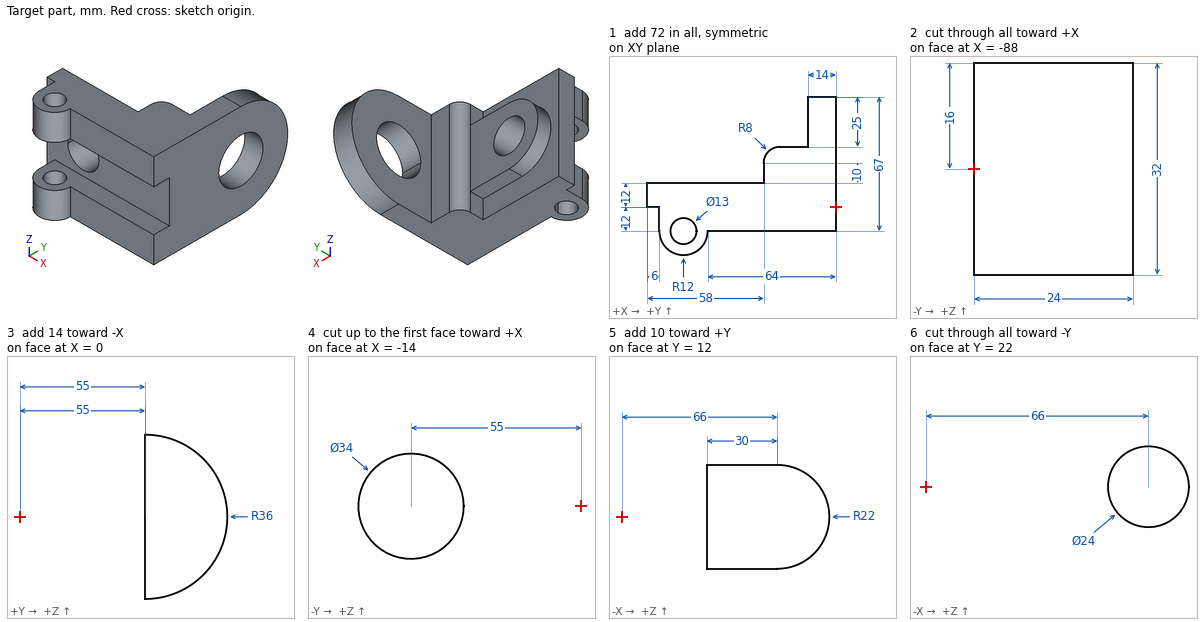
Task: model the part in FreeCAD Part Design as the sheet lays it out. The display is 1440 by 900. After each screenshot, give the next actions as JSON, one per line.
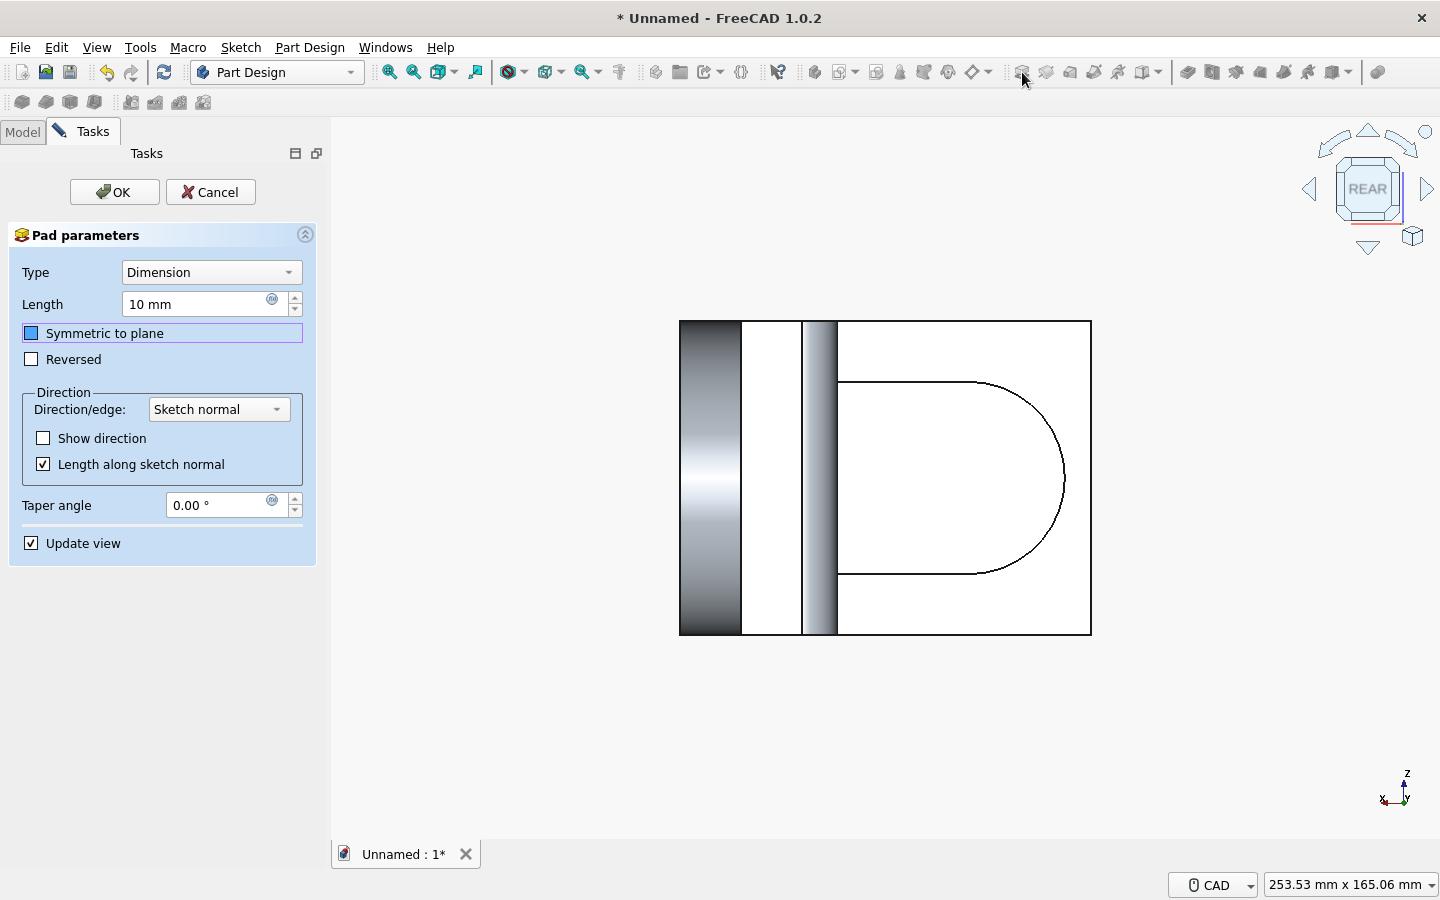
{"action": "left_click", "coordinate": [115, 192]}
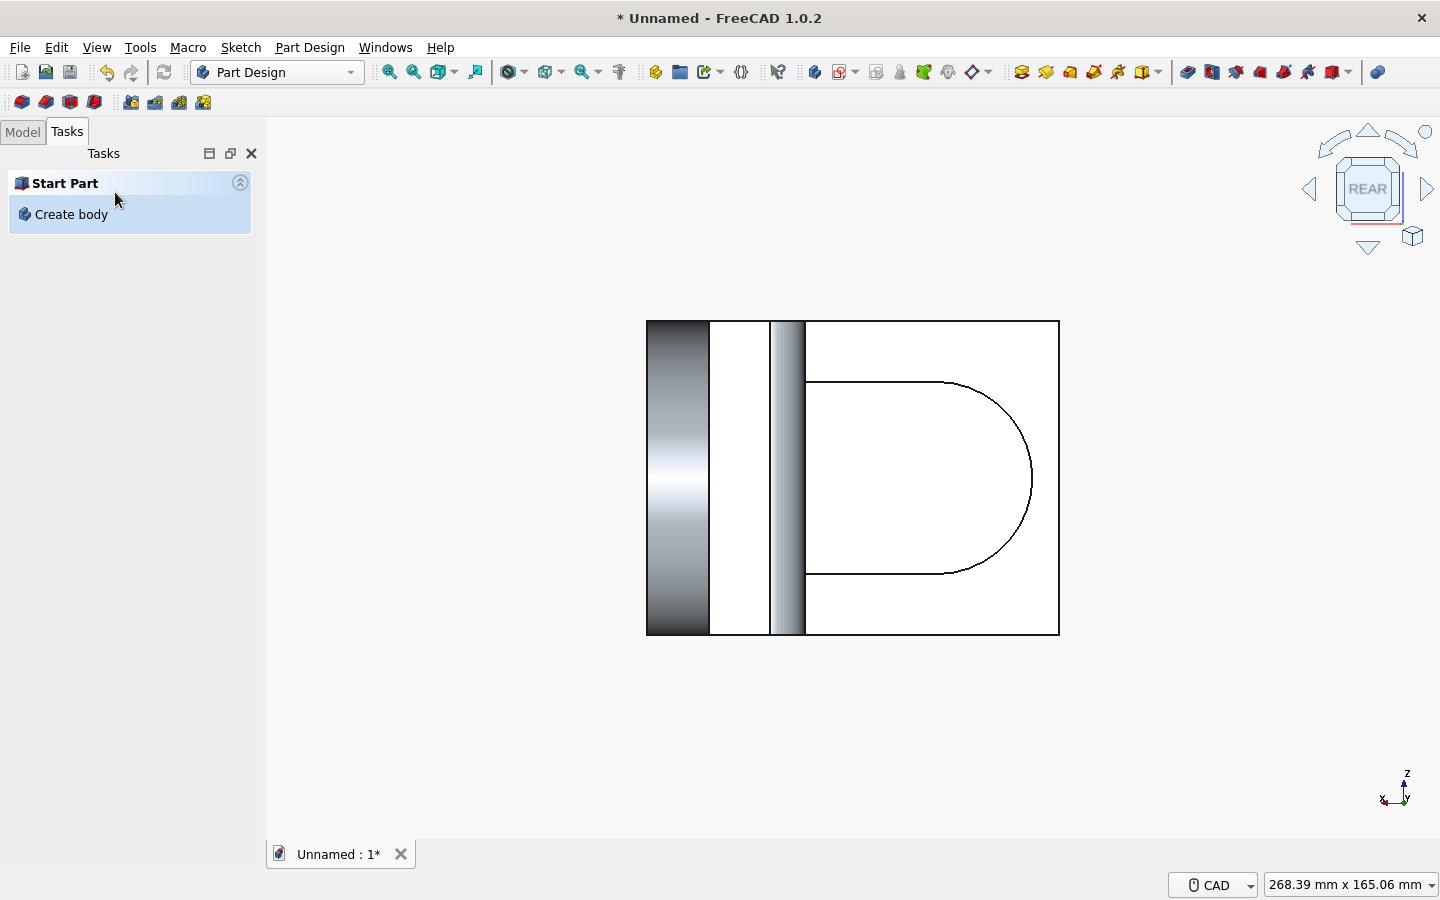
{"action": "left_click", "coordinate": [390, 72]}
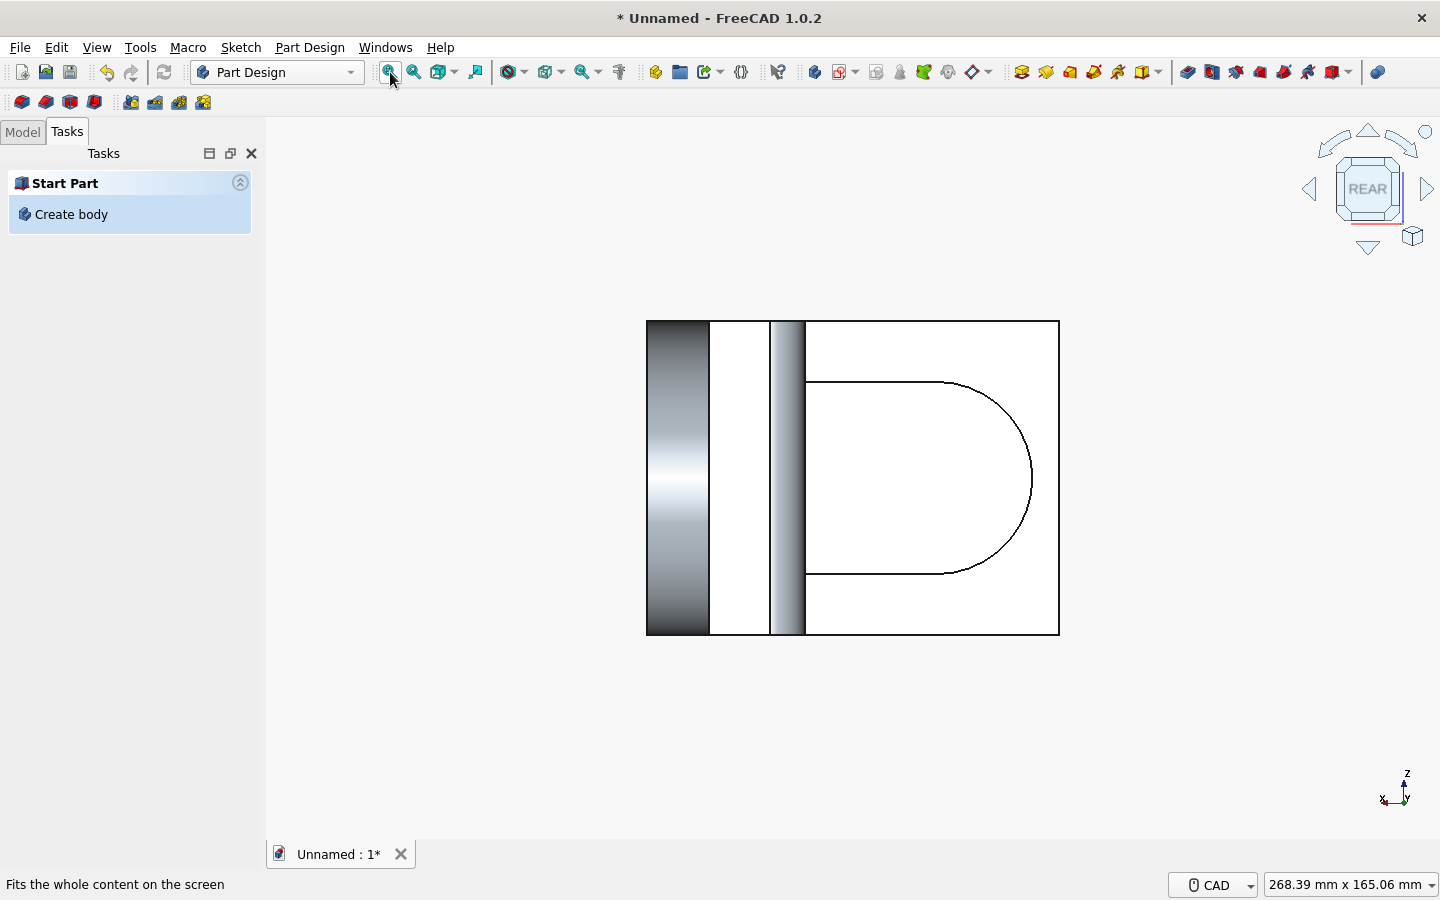
{"action": "left_click", "coordinate": [919, 477]}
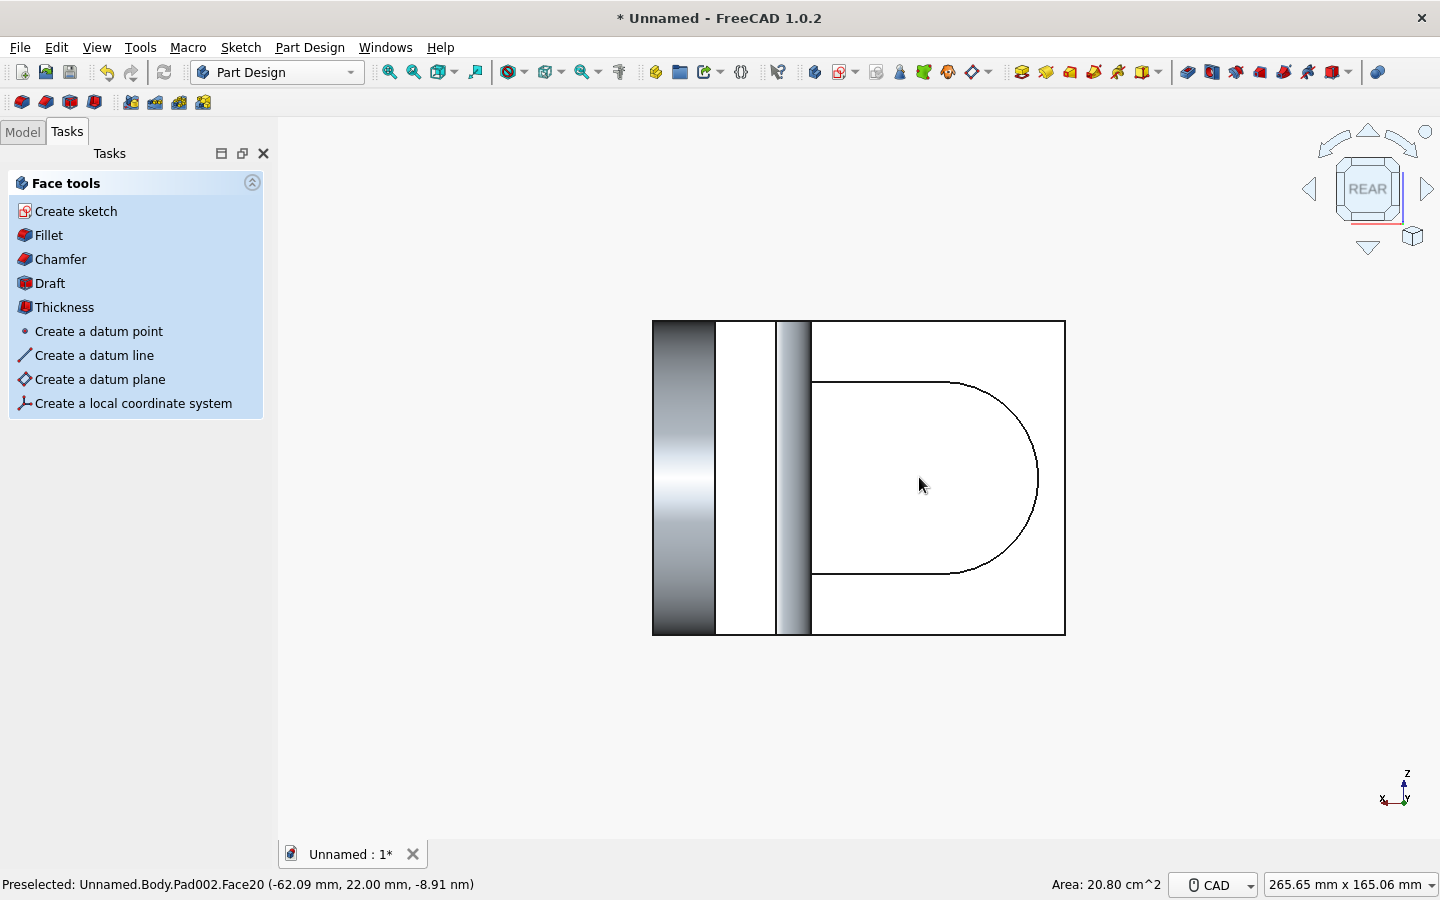
{"action": "left_click", "coordinate": [840, 72]}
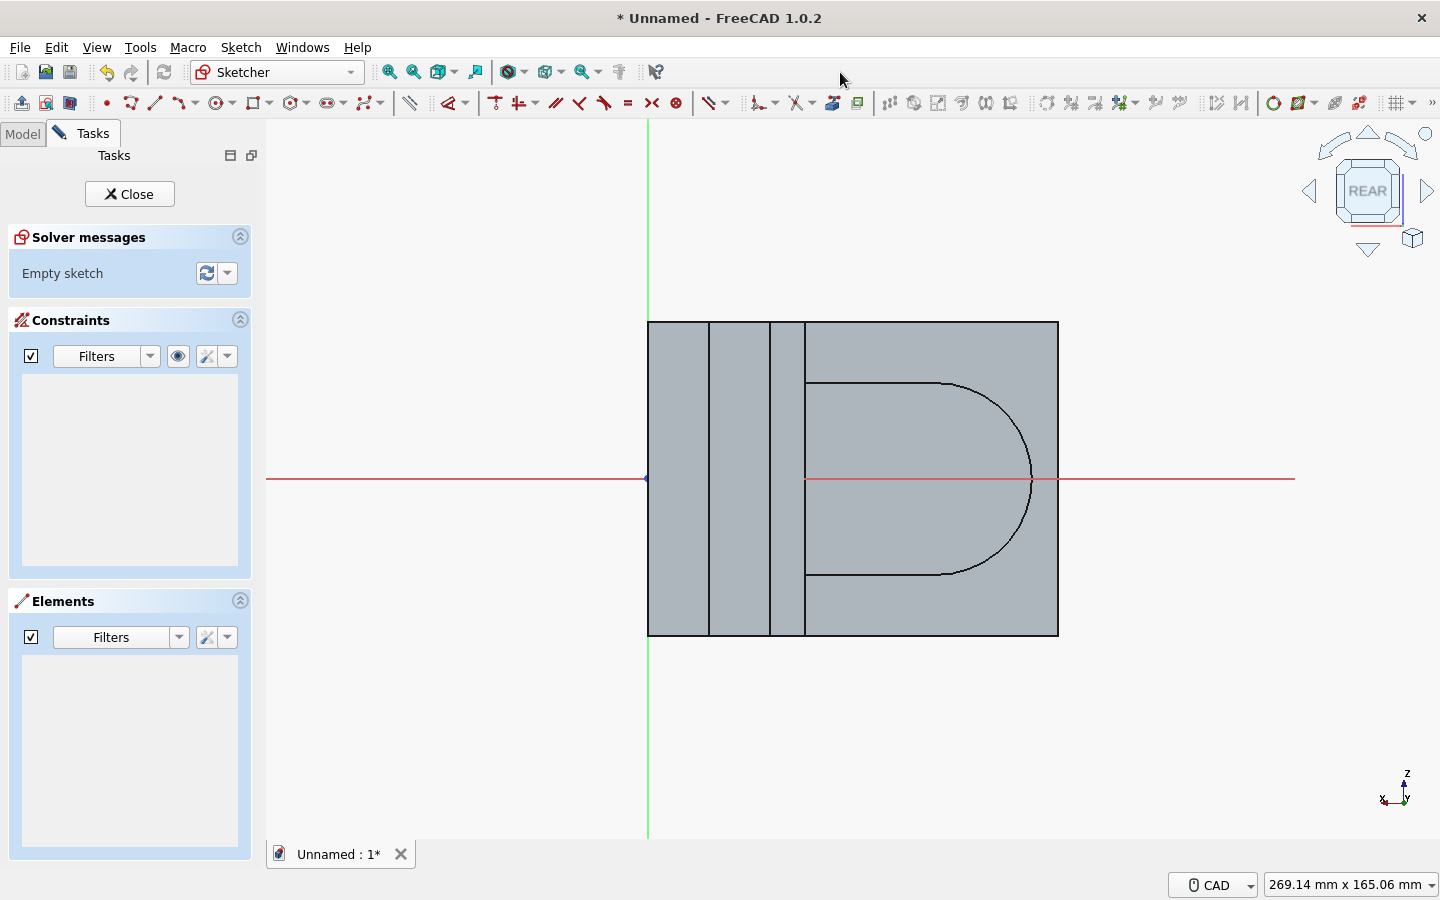
{"action": "scroll", "coordinate": [985, 479], "scroll_direction": "up", "scroll_amount": 7}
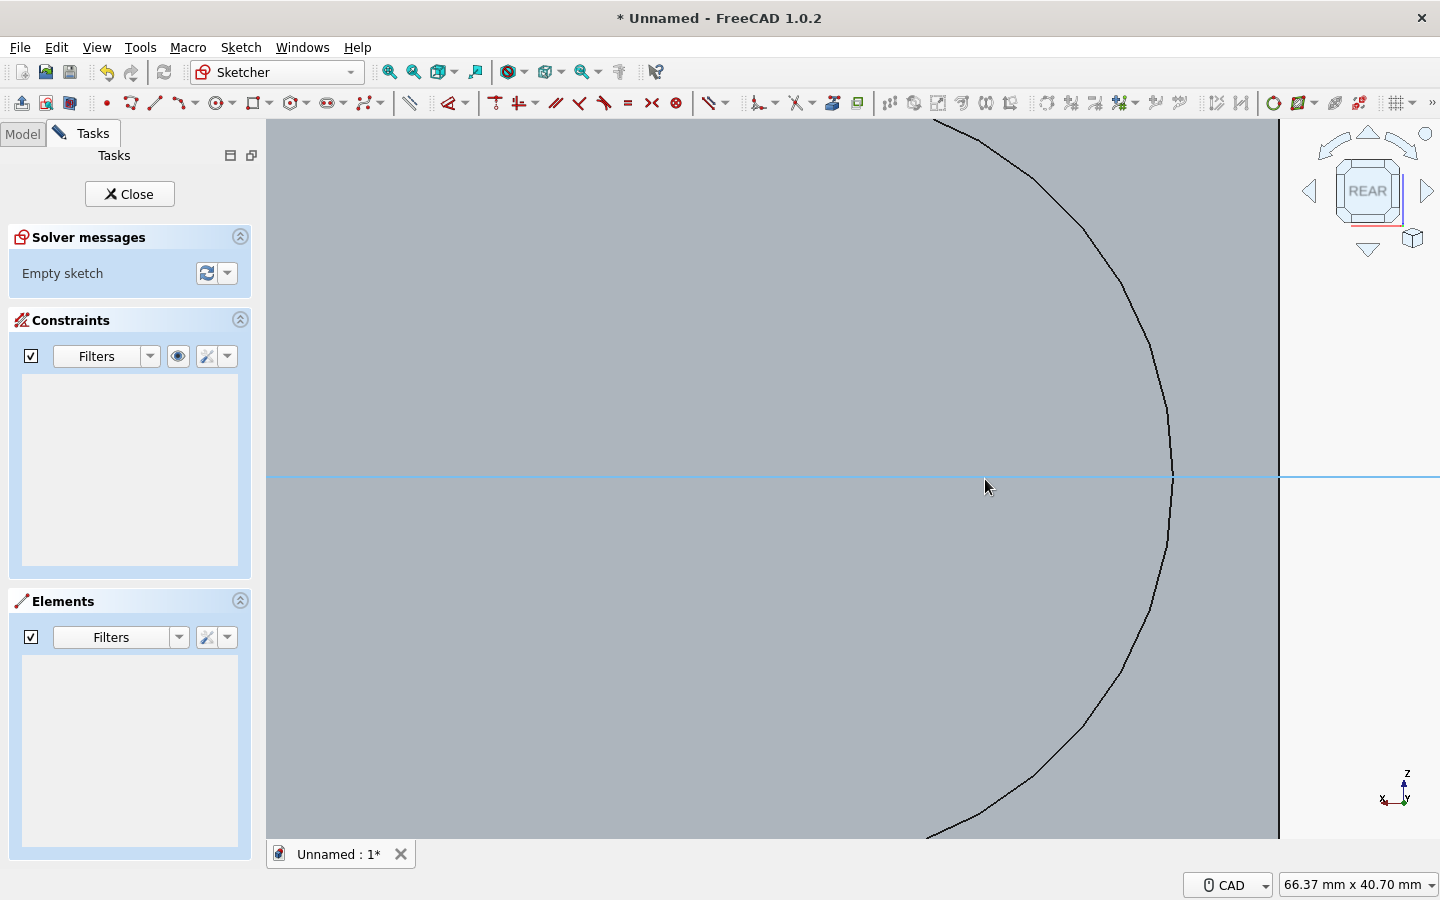
{"action": "left_click", "coordinate": [216, 104]}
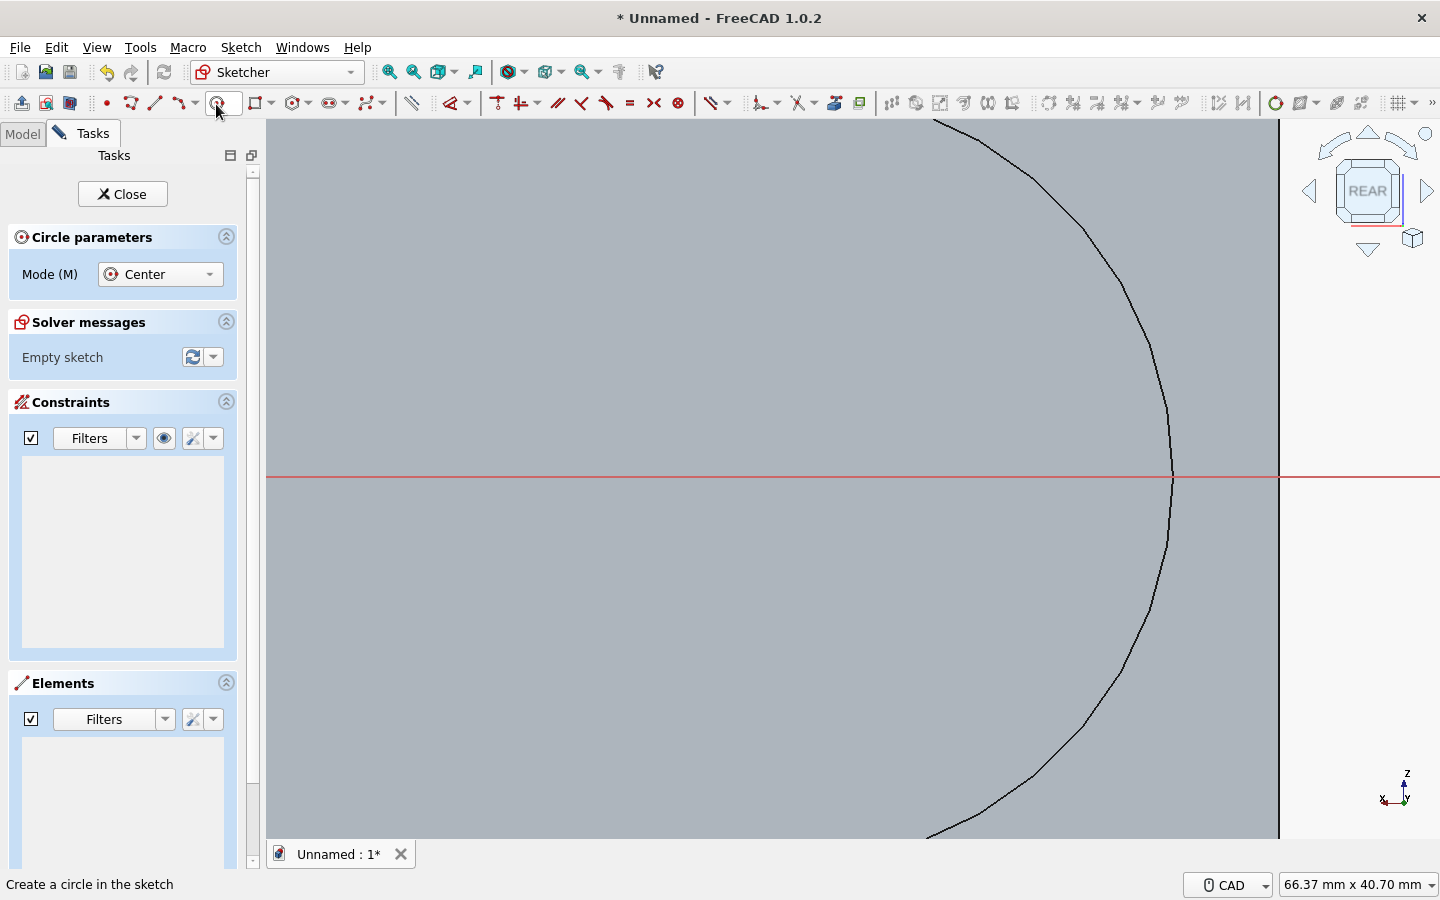
{"action": "left_click", "coordinate": [784, 477]}
{"action": "mouse_move", "coordinate": [934, 327]}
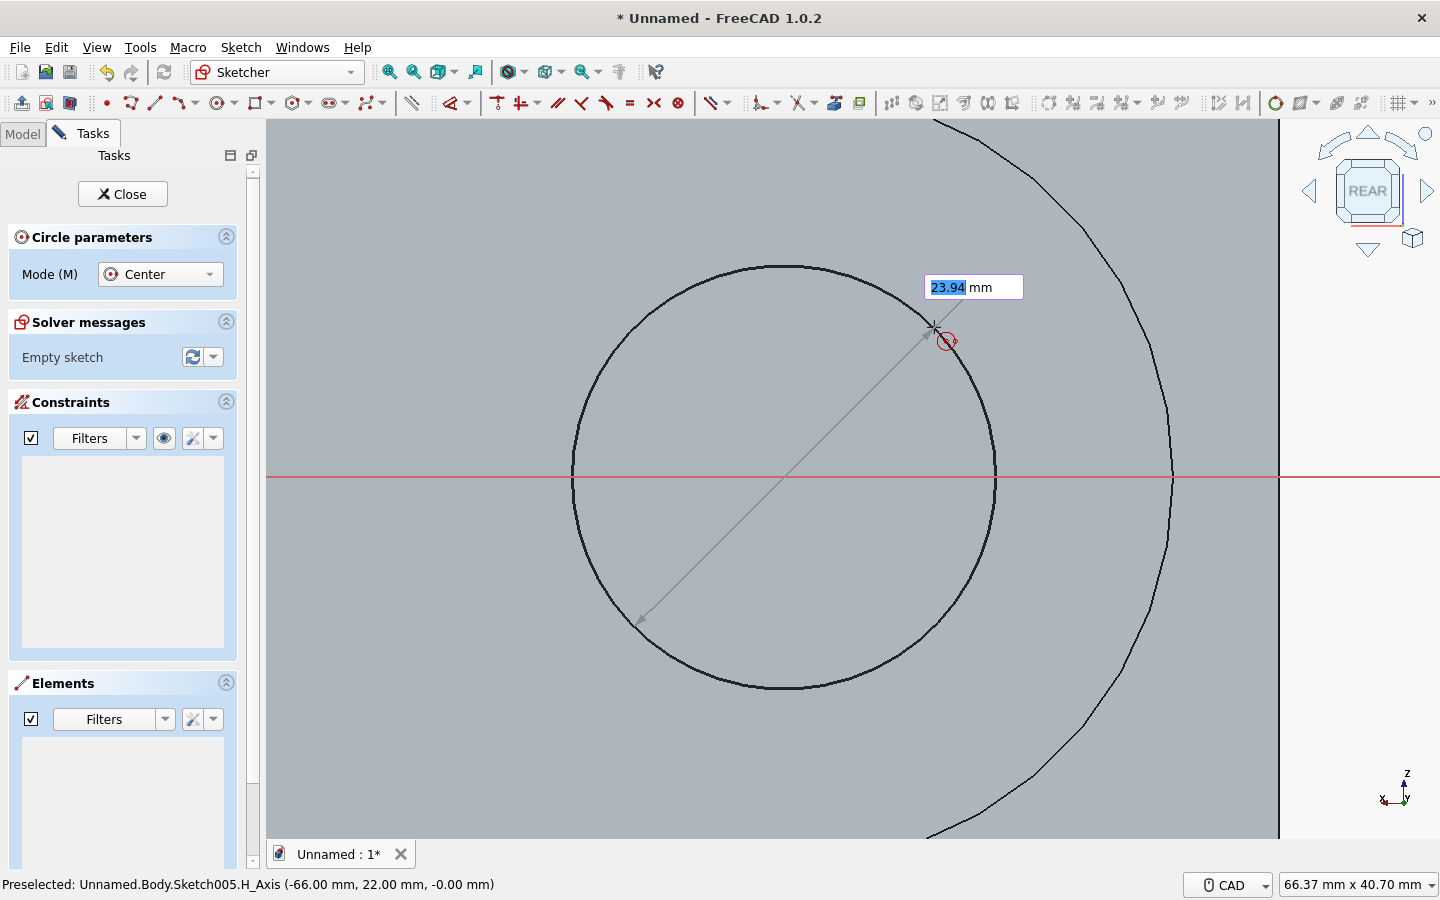
{"action": "type", "text": "24"}
{"action": "key", "text": "Return"}
{"action": "key", "text": "Escape"}